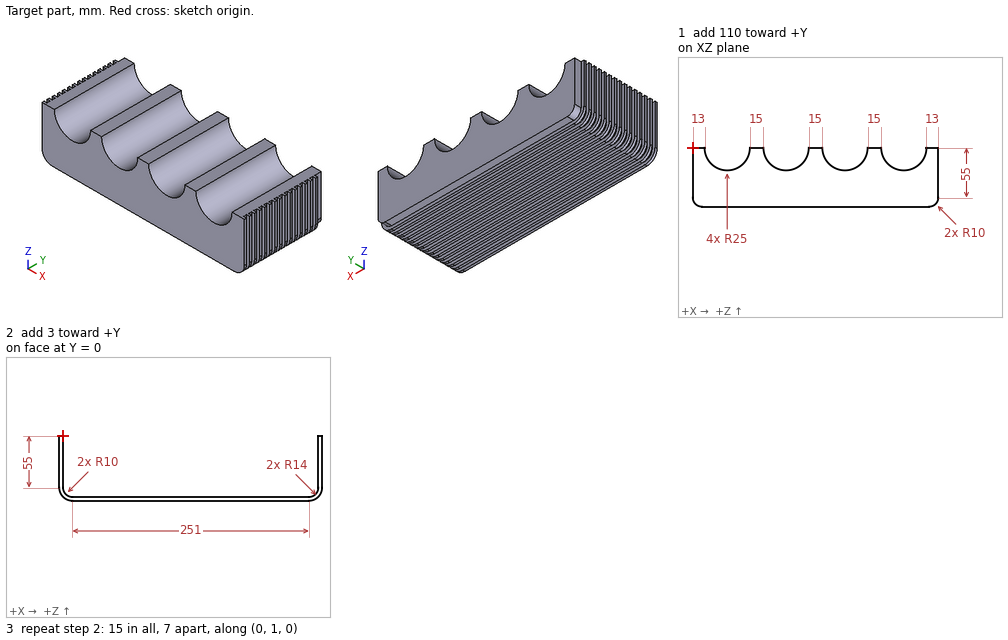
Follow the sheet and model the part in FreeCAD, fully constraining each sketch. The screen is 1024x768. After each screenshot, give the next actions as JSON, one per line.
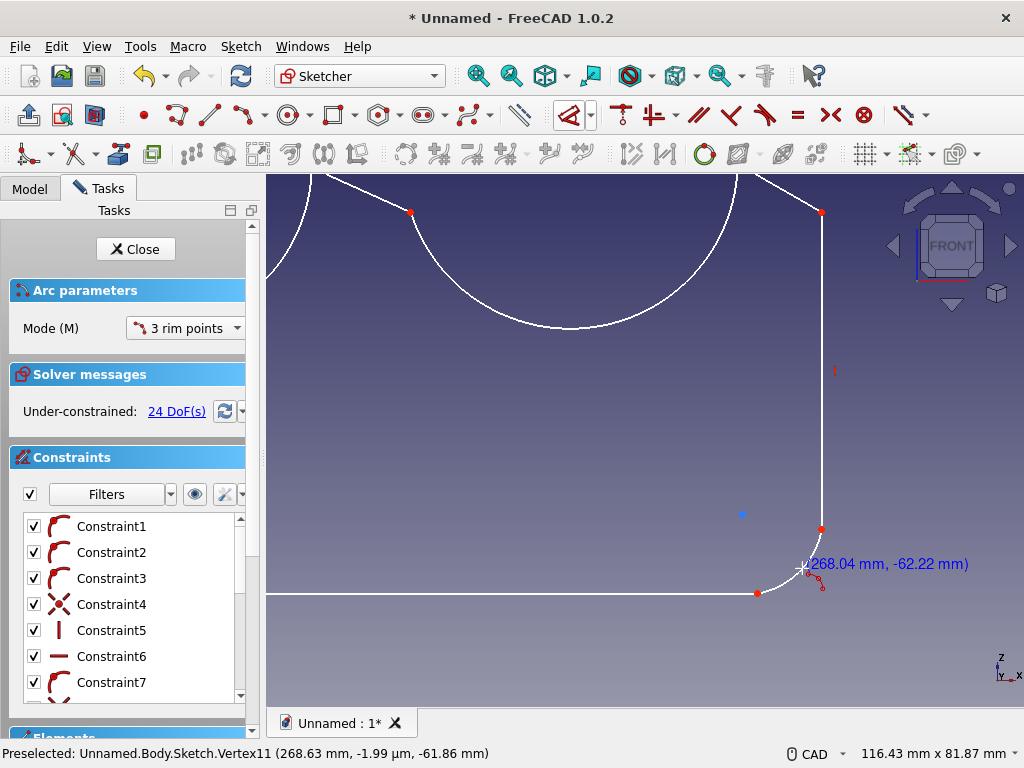
{"action": "scroll", "coordinate": [785, 462], "scroll_direction": "down", "scroll_amount": 7}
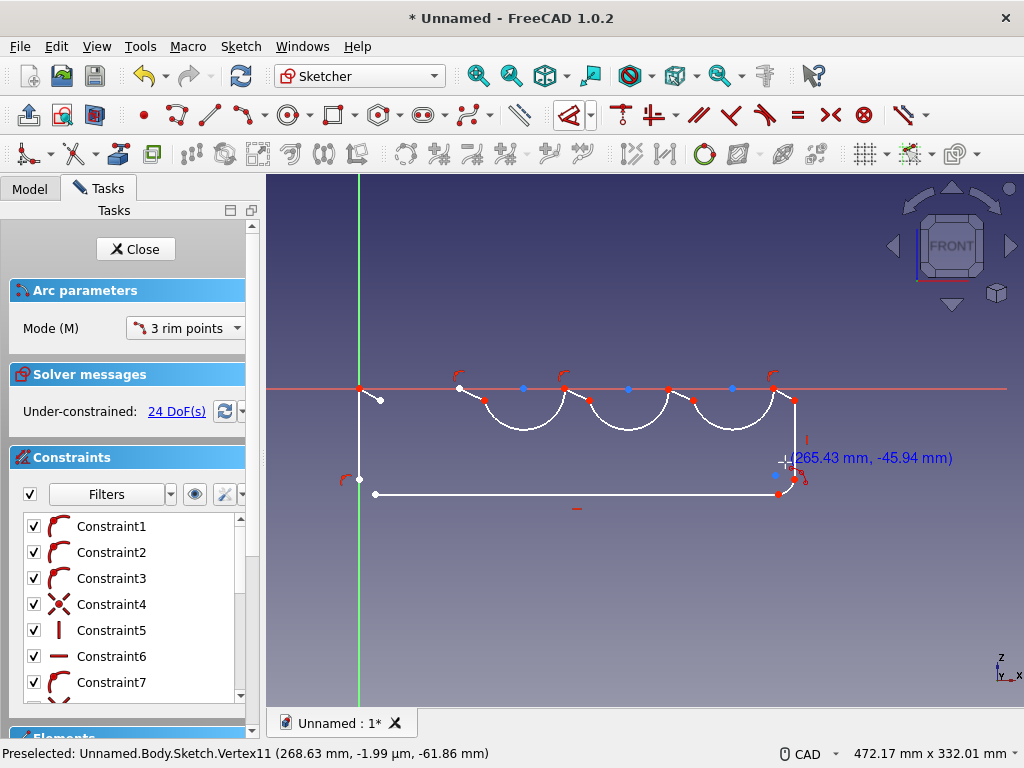
{"action": "left_click", "coordinate": [376, 495]}
{"action": "left_click", "coordinate": [359, 479]}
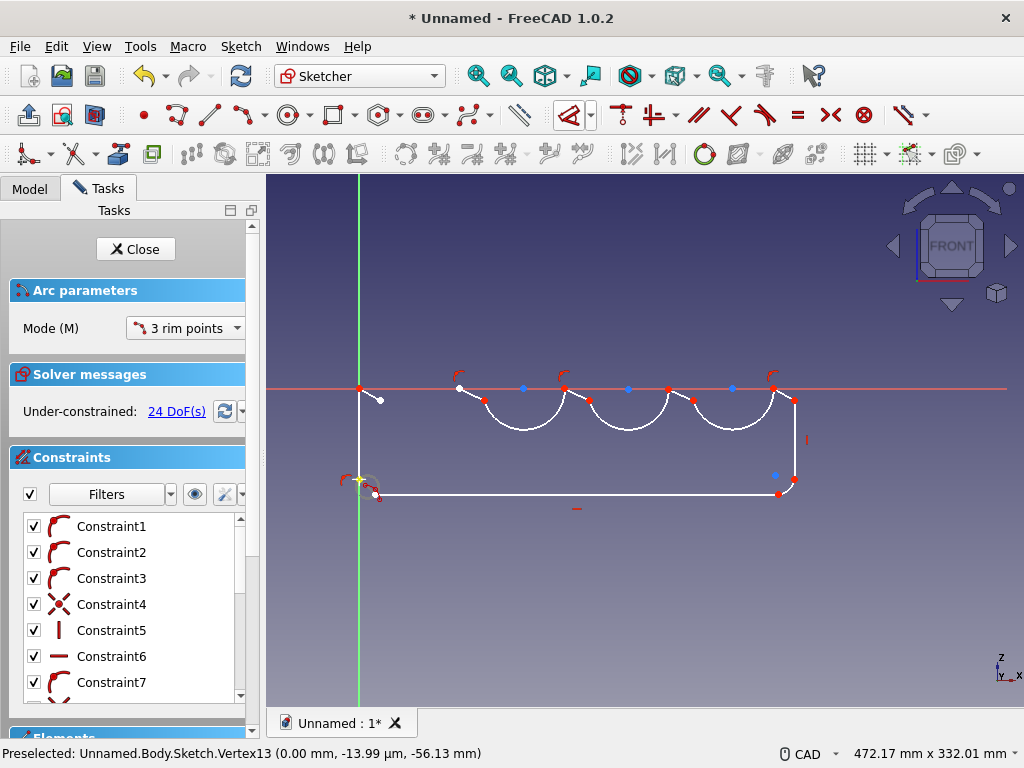
{"action": "scroll", "coordinate": [364, 489], "scroll_direction": "up", "scroll_amount": 7}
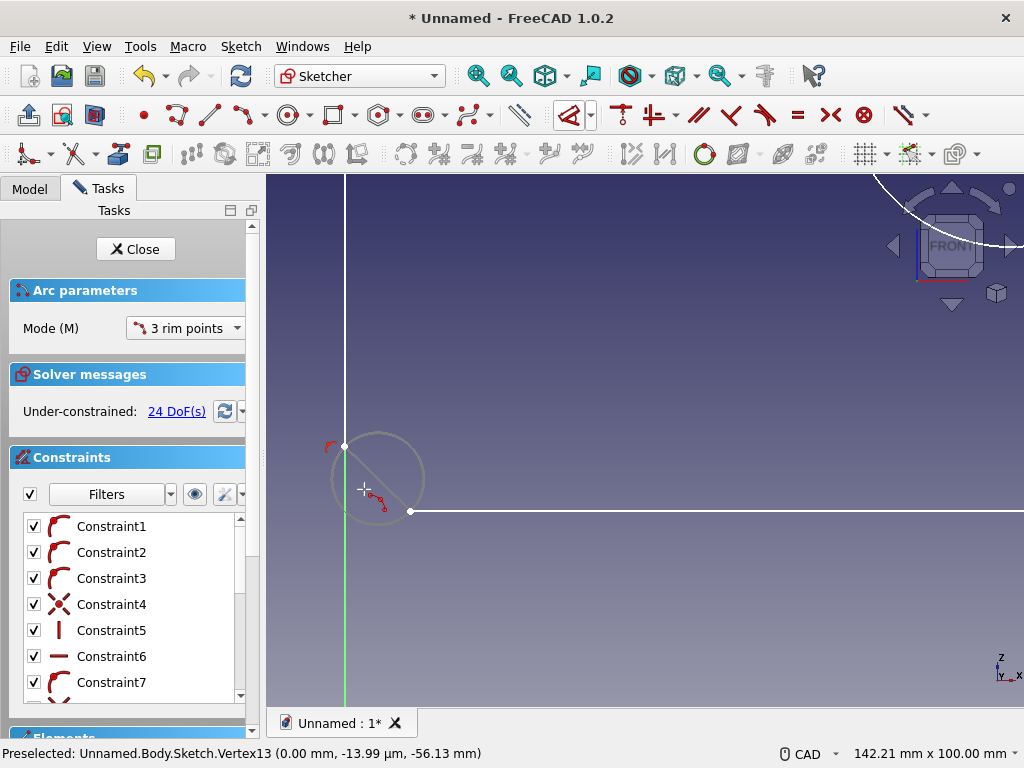
{"action": "left_click", "coordinate": [364, 485]}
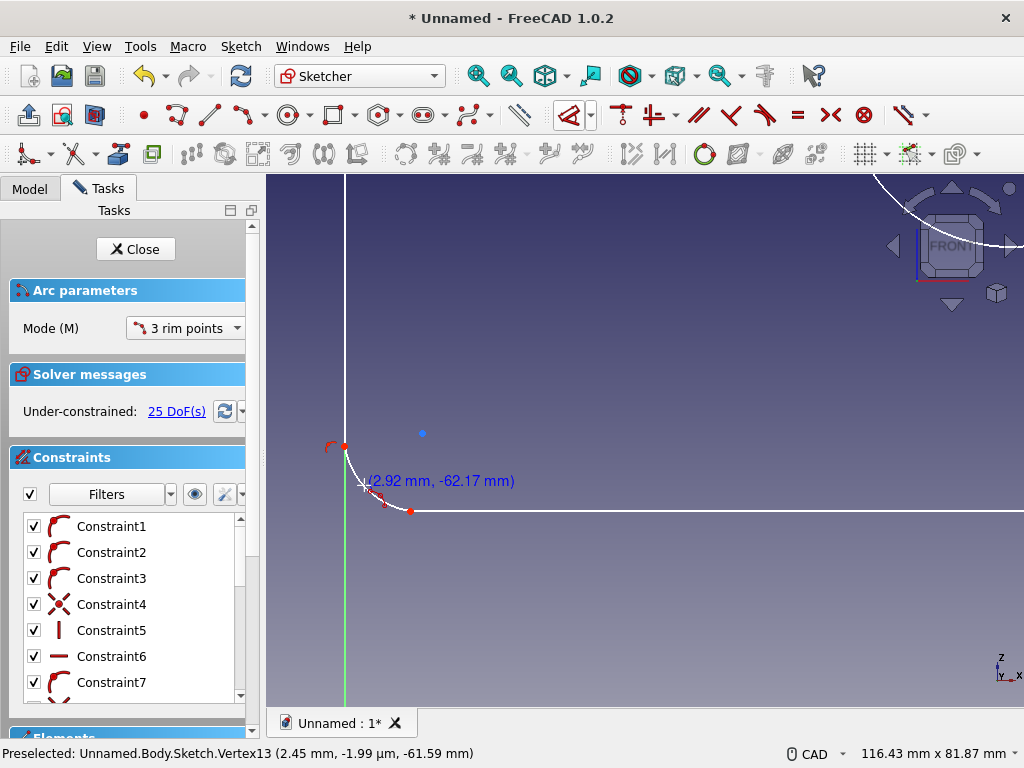
{"action": "scroll", "coordinate": [364, 489], "scroll_direction": "down", "scroll_amount": 7}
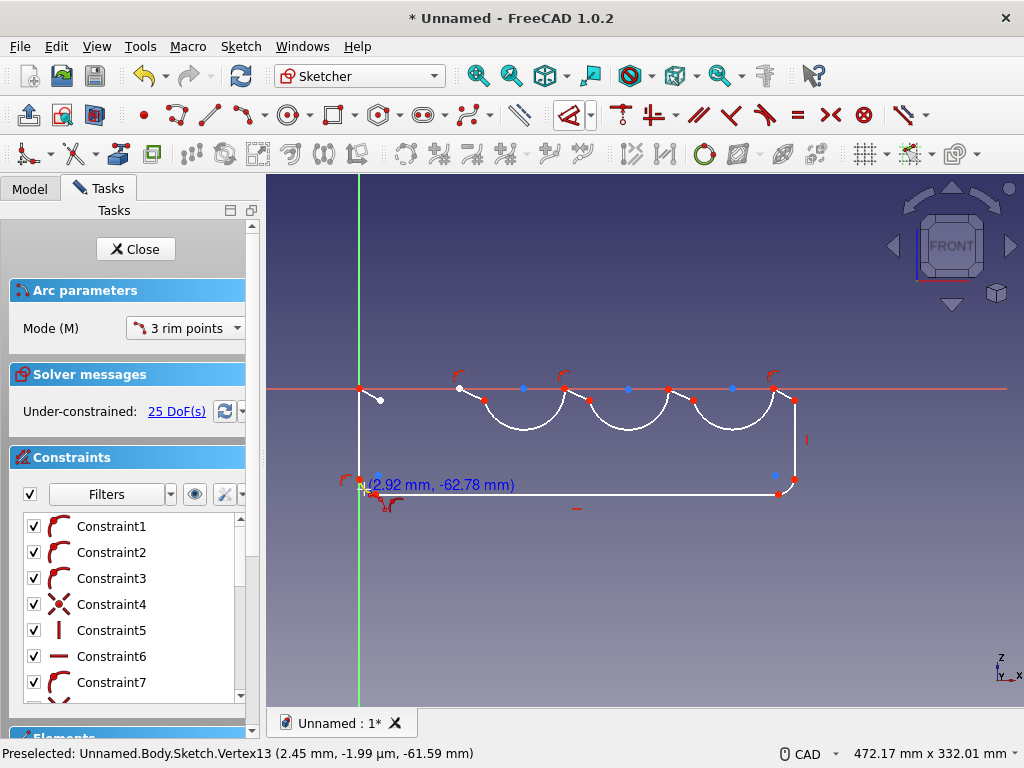
{"action": "scroll", "coordinate": [380, 389], "scroll_direction": "up", "scroll_amount": 3}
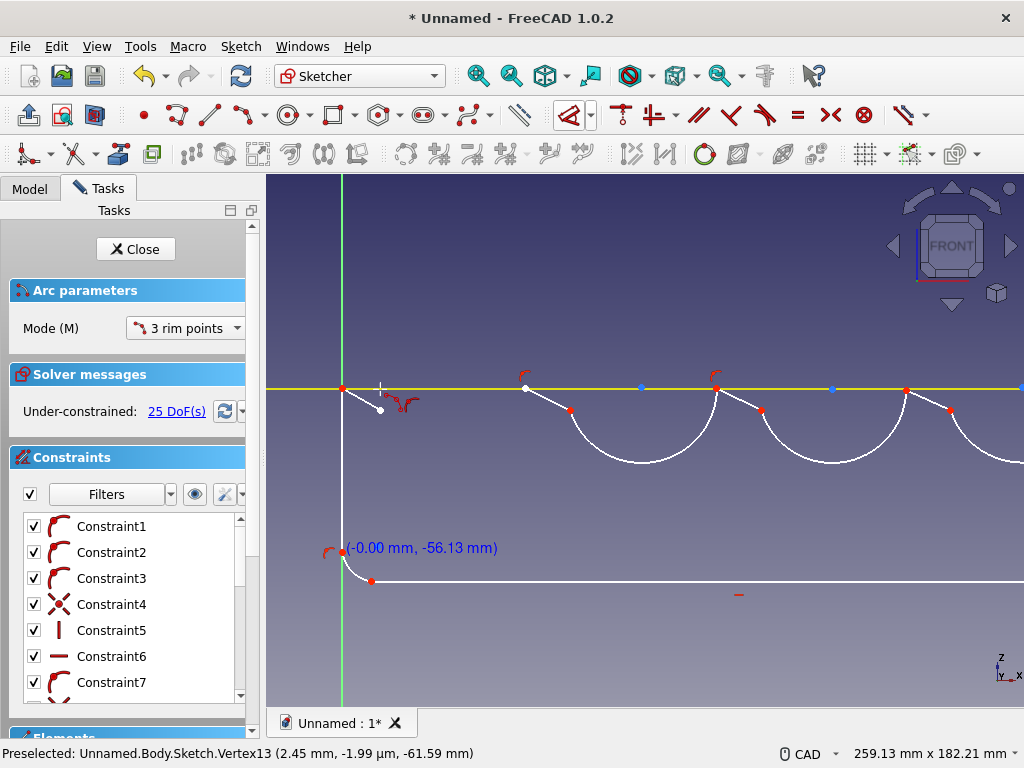
{"action": "left_click", "coordinate": [381, 410]}
{"action": "left_click", "coordinate": [526, 388]}
{"action": "left_click", "coordinate": [454, 462]}
{"action": "key", "text": "Escape"}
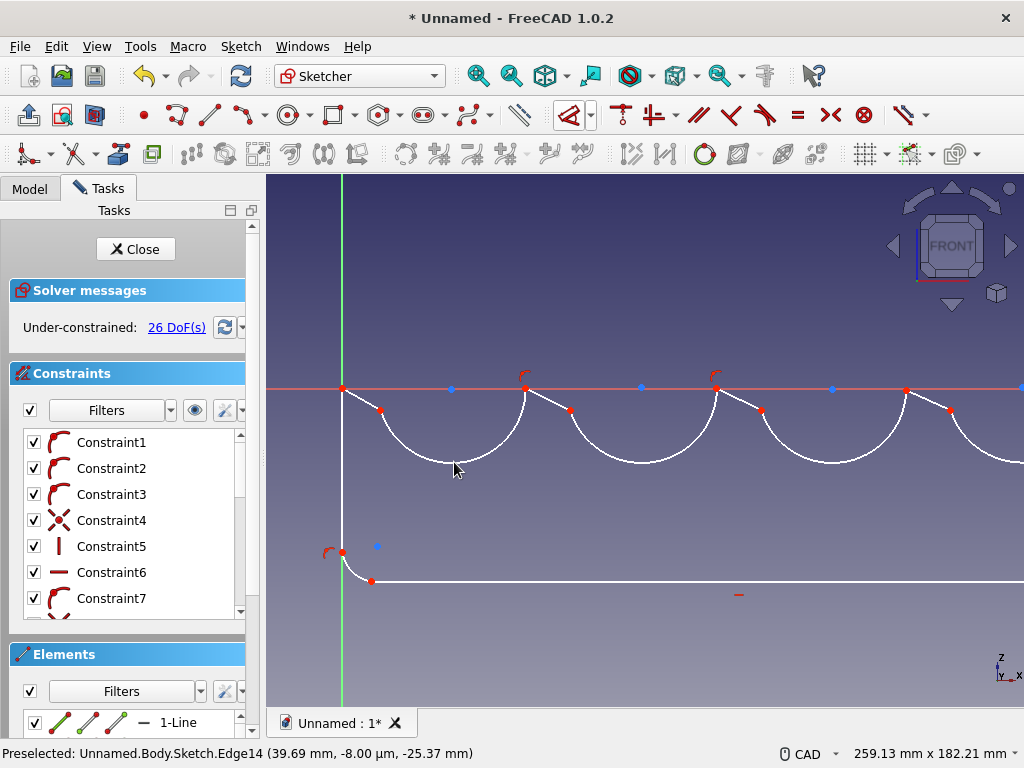
{"action": "scroll", "coordinate": [379, 388], "scroll_direction": "down", "scroll_amount": 3}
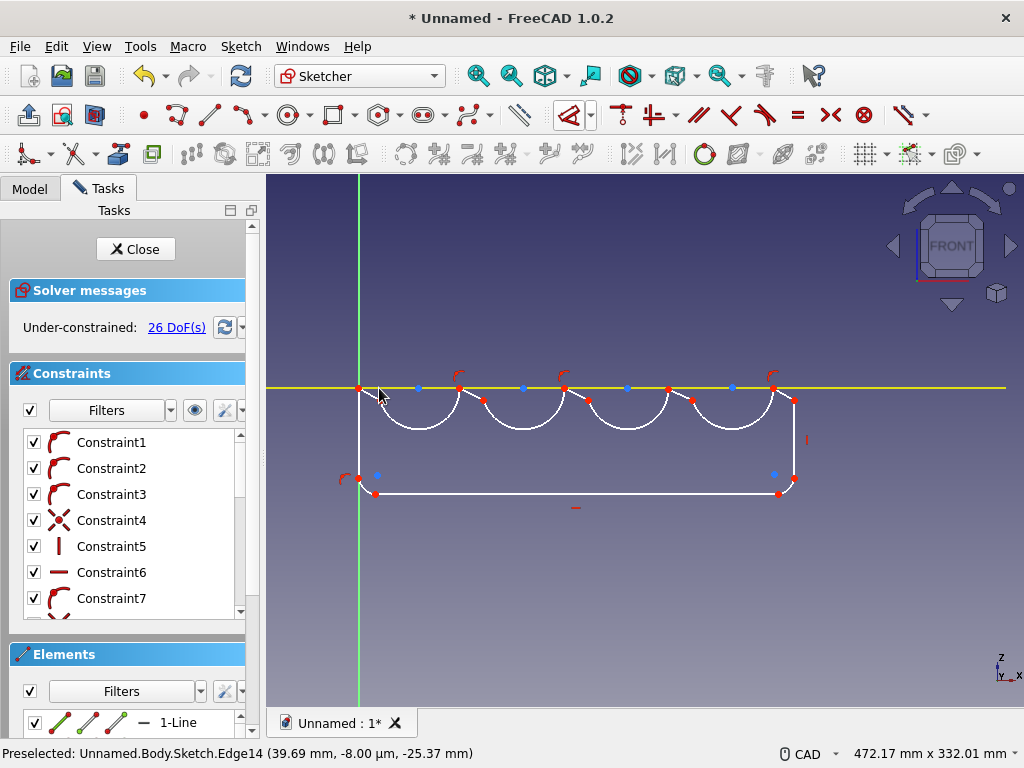
{"action": "left_click", "coordinate": [794, 424]}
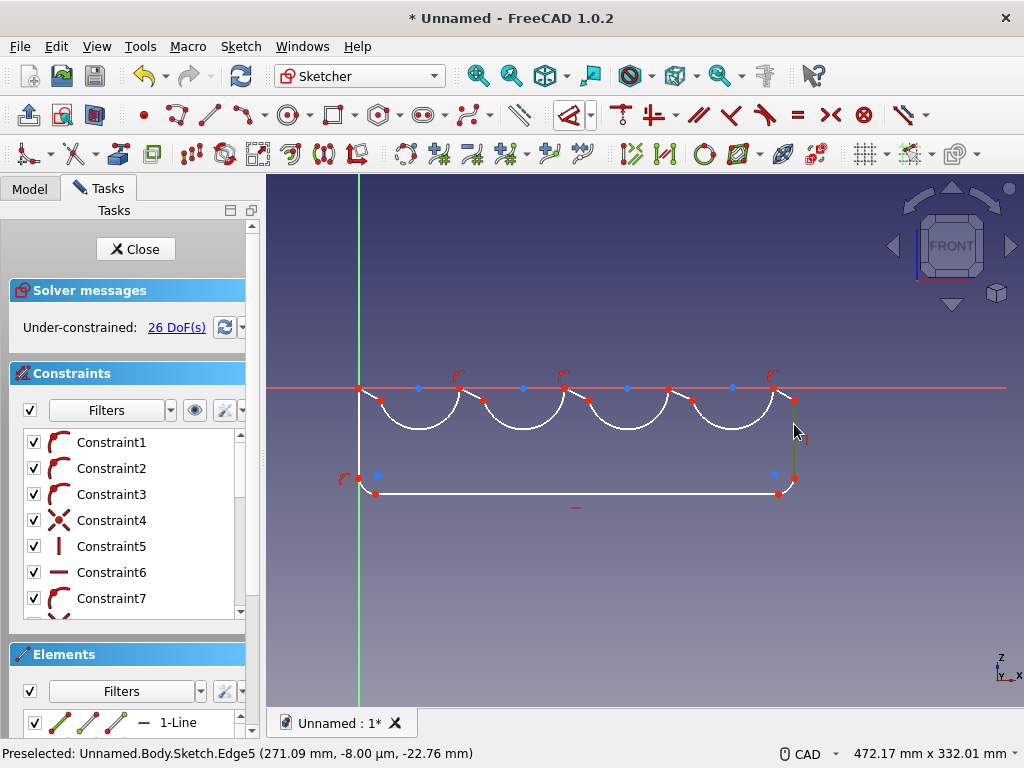
{"action": "left_click", "coordinate": [789, 489]}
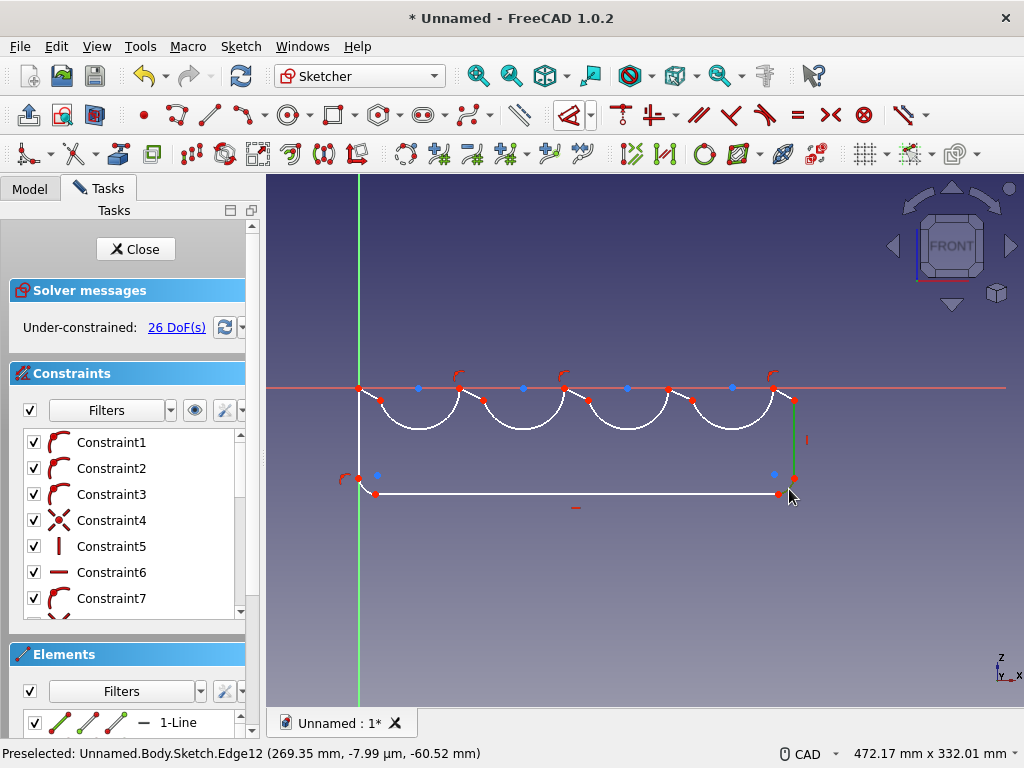
{"action": "left_click", "coordinate": [765, 116]}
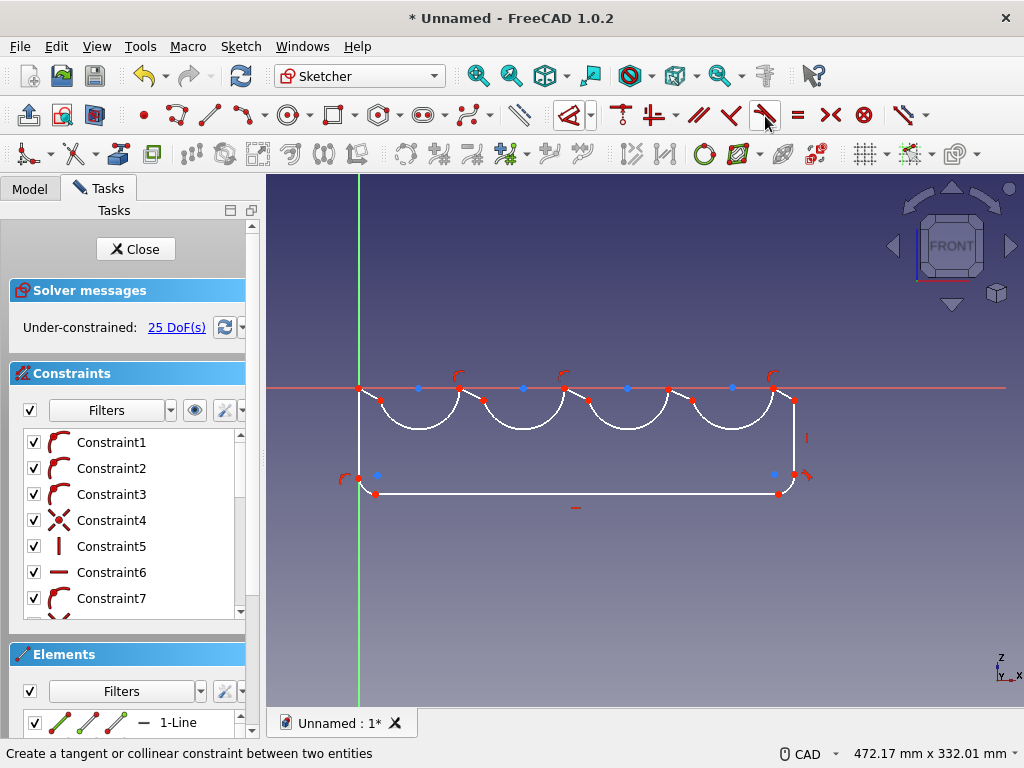
{"action": "left_click", "coordinate": [657, 494]}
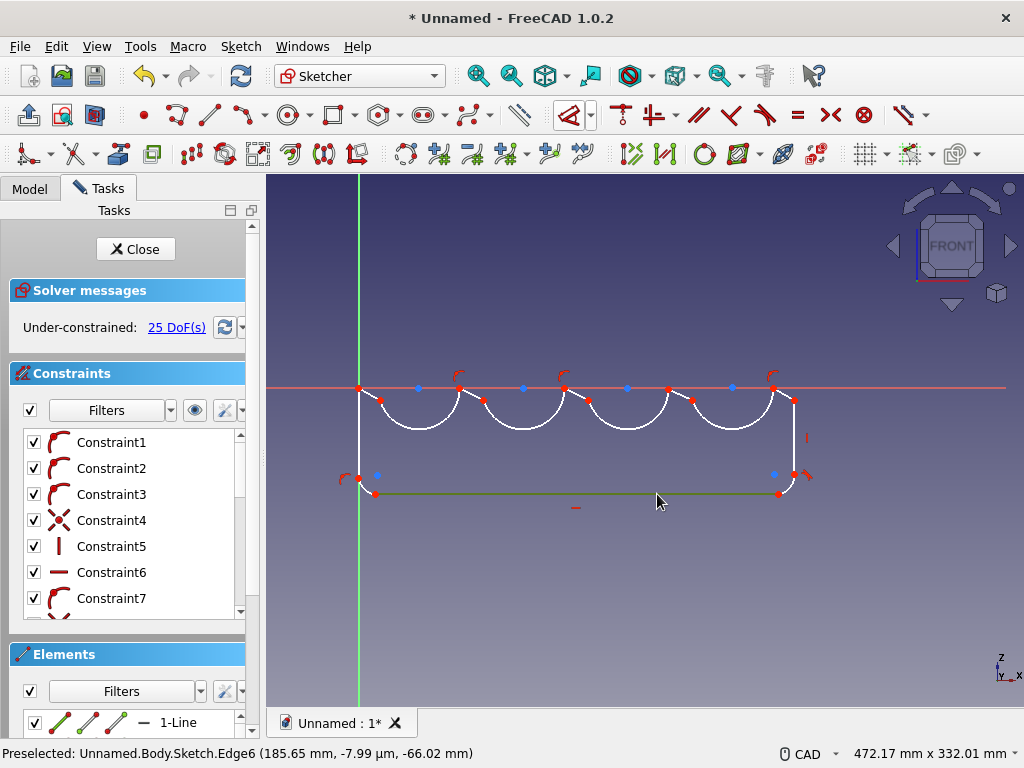
{"action": "left_click", "coordinate": [790, 488]}